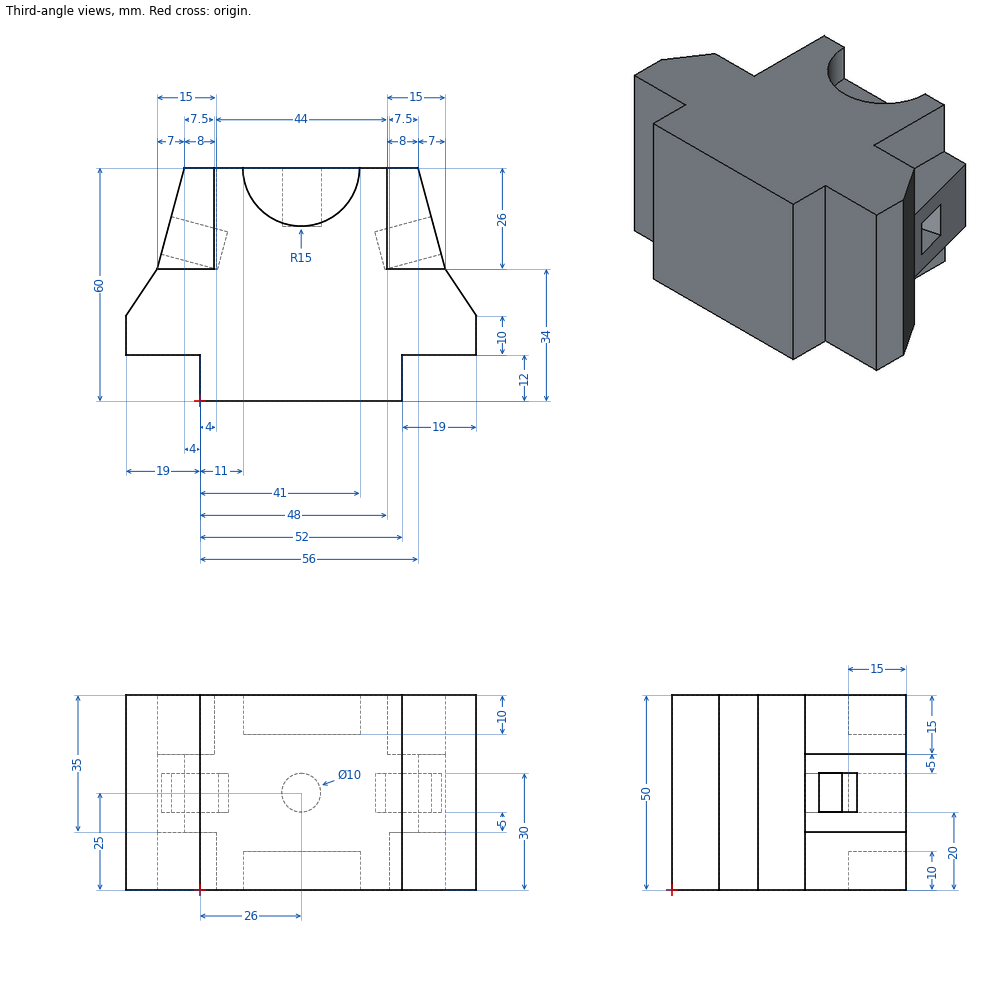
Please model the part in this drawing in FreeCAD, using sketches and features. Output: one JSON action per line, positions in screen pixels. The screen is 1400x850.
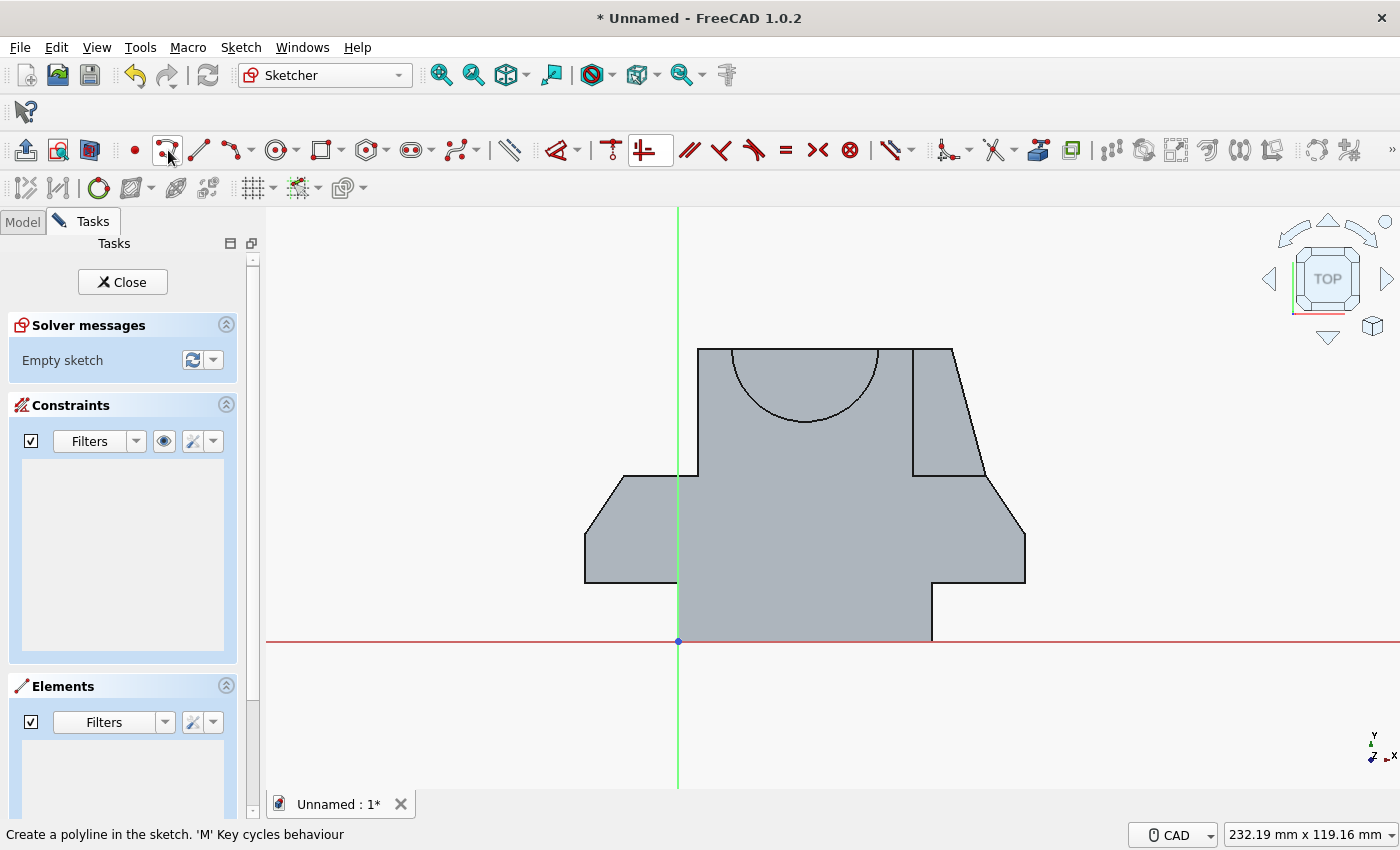
{"action": "left_click", "coordinate": [698, 476]}
{"action": "left_click", "coordinate": [698, 349]}
{"action": "left_click", "coordinate": [659, 349]}
{"action": "left_click", "coordinate": [624, 476]}
{"action": "left_click", "coordinate": [698, 477]}
{"action": "key", "text": "Escape"}
{"action": "key", "text": "Escape"}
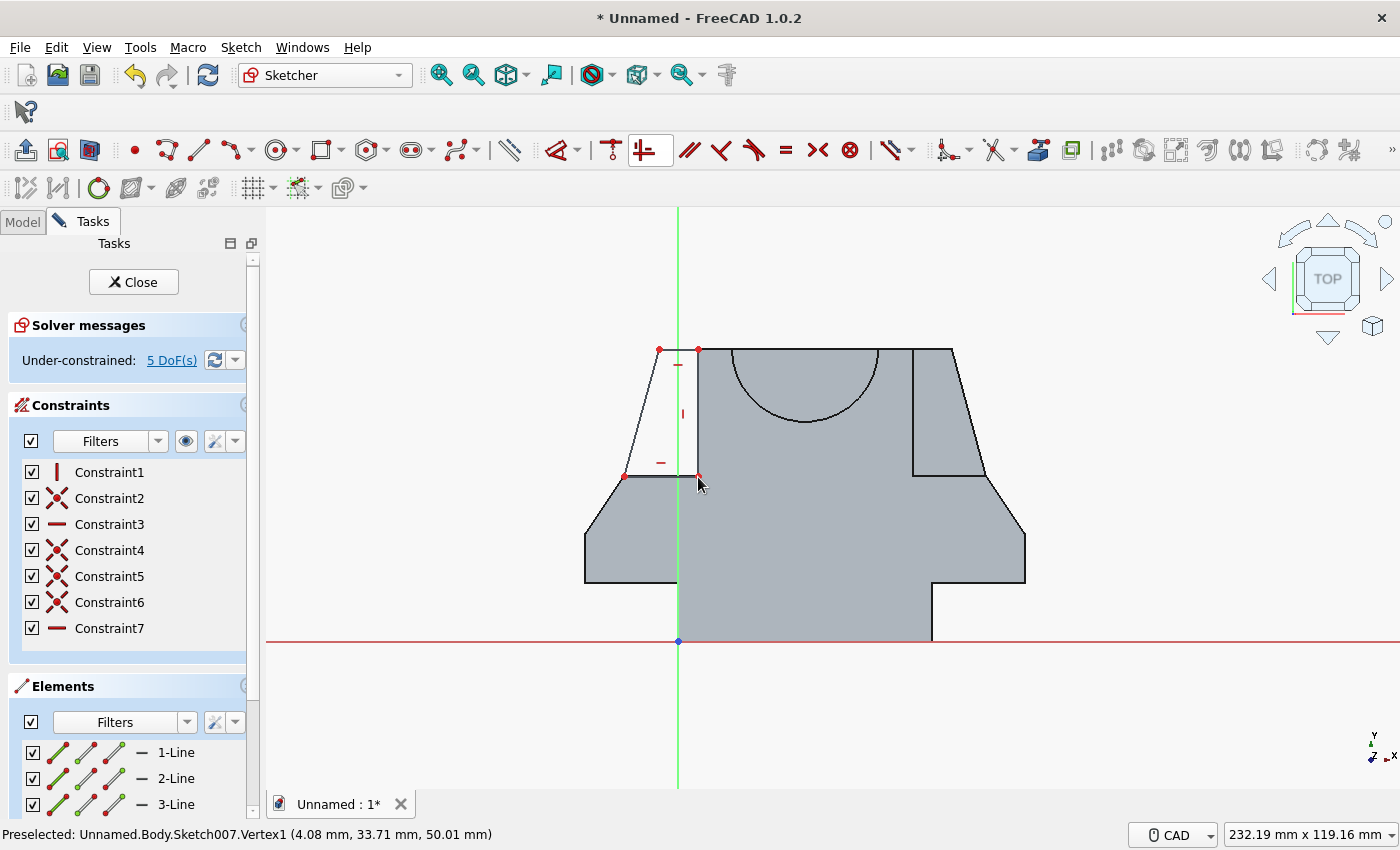
{"action": "left_click", "coordinate": [556, 150]}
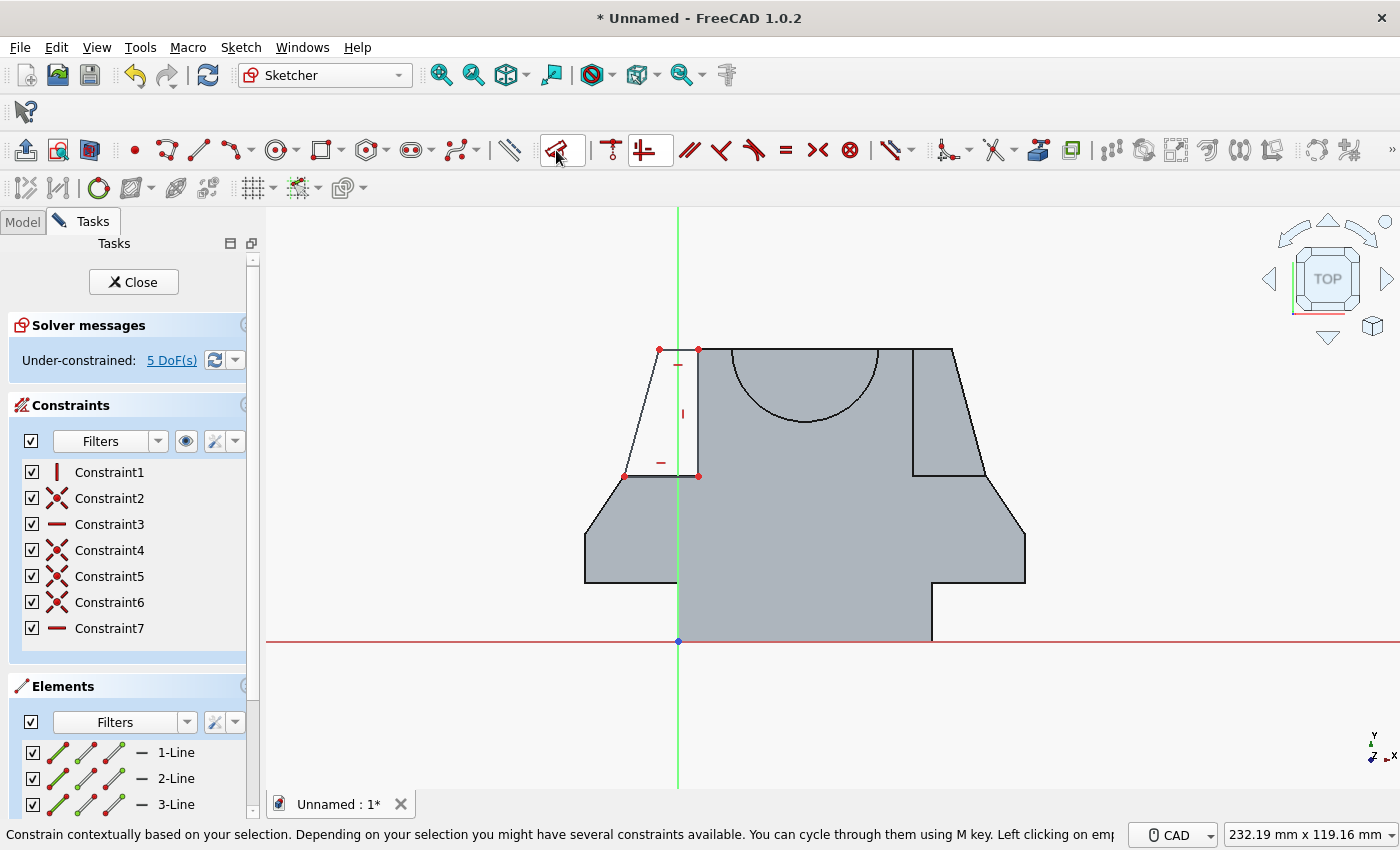
{"action": "left_click", "coordinate": [675, 350]}
{"action": "left_click", "coordinate": [665, 316]}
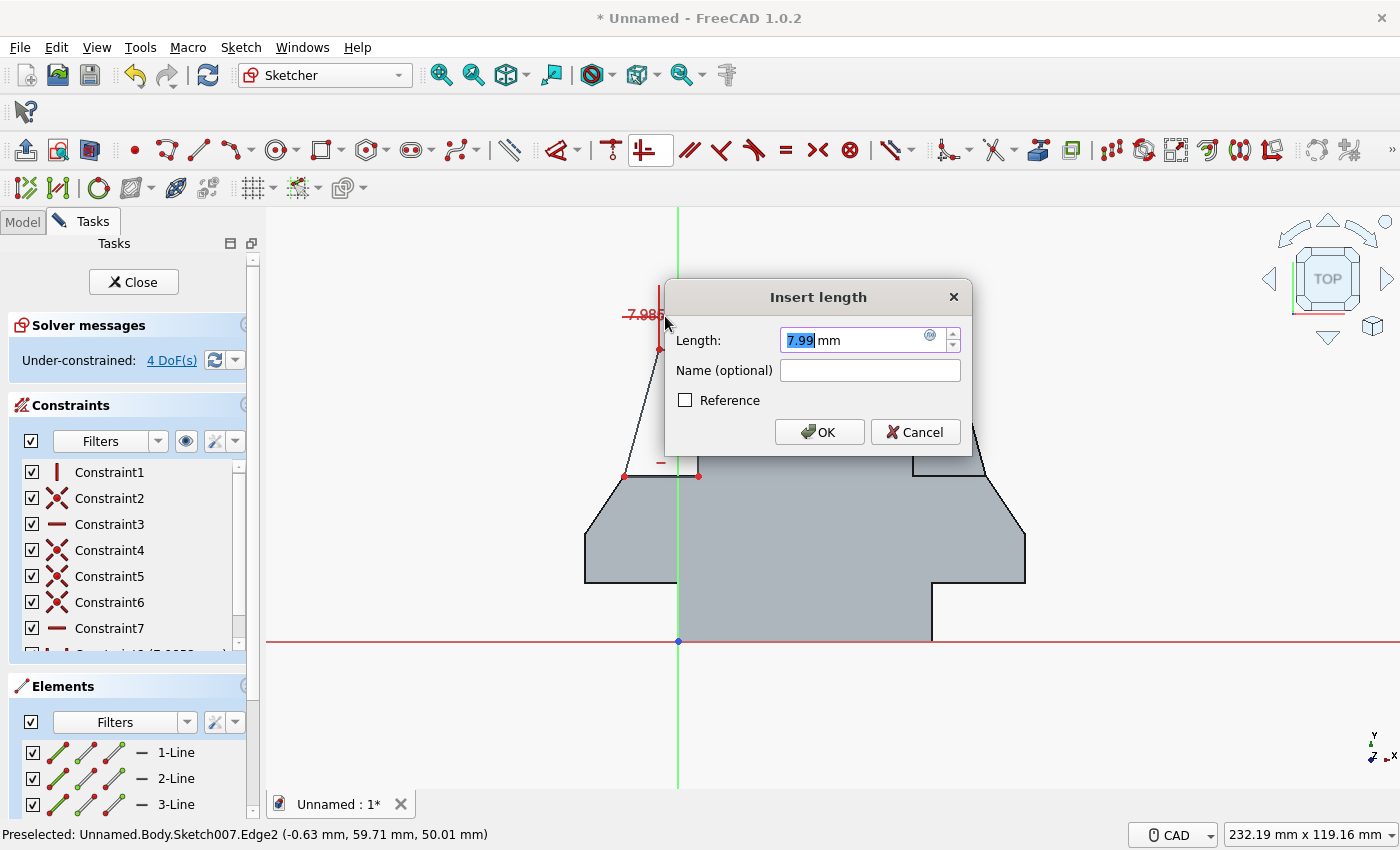
{"action": "type", "text": "8"}
{"action": "key", "text": "Return"}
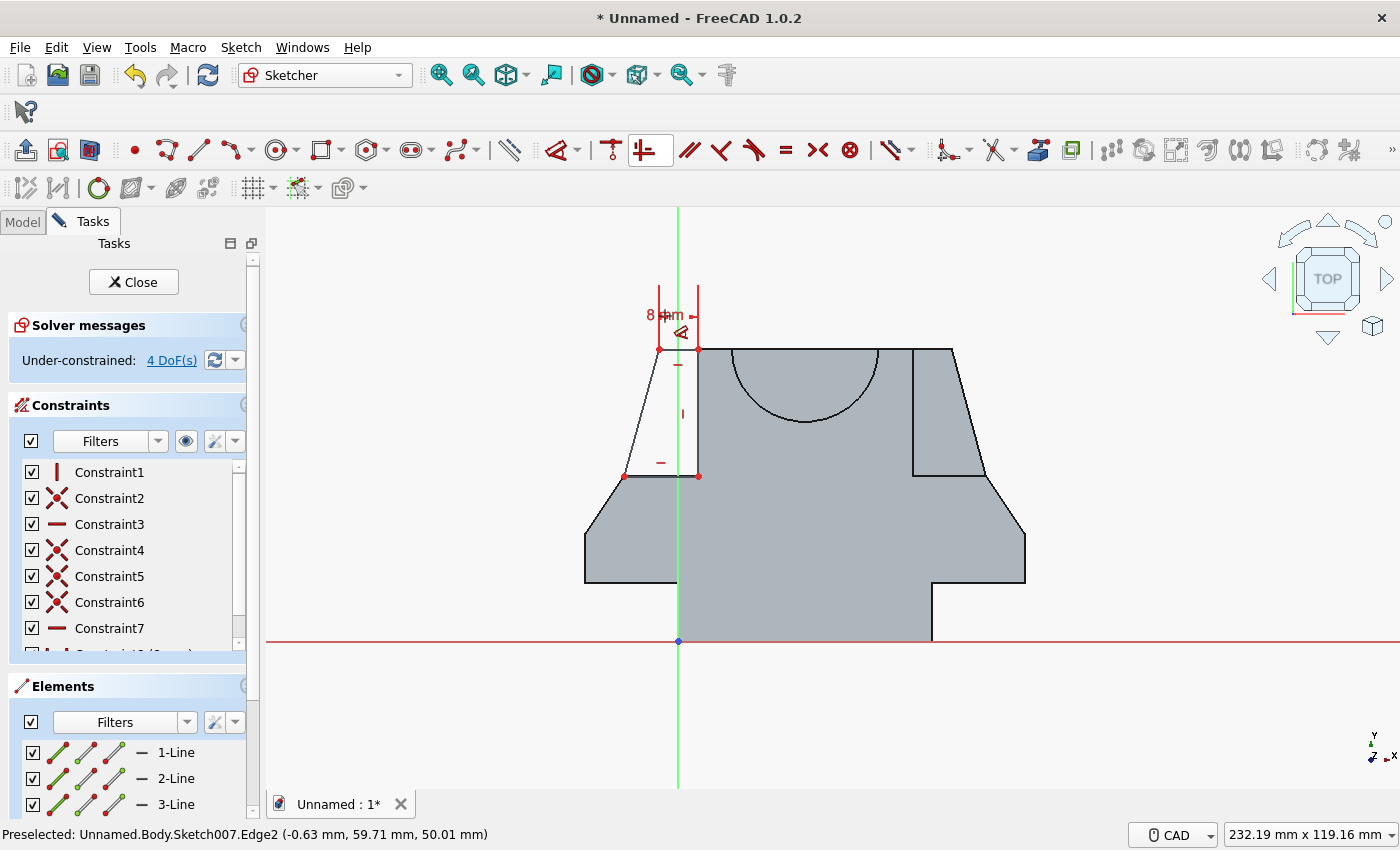
{"action": "left_click", "coordinate": [698, 439]}
{"action": "left_click", "coordinate": [732, 414]}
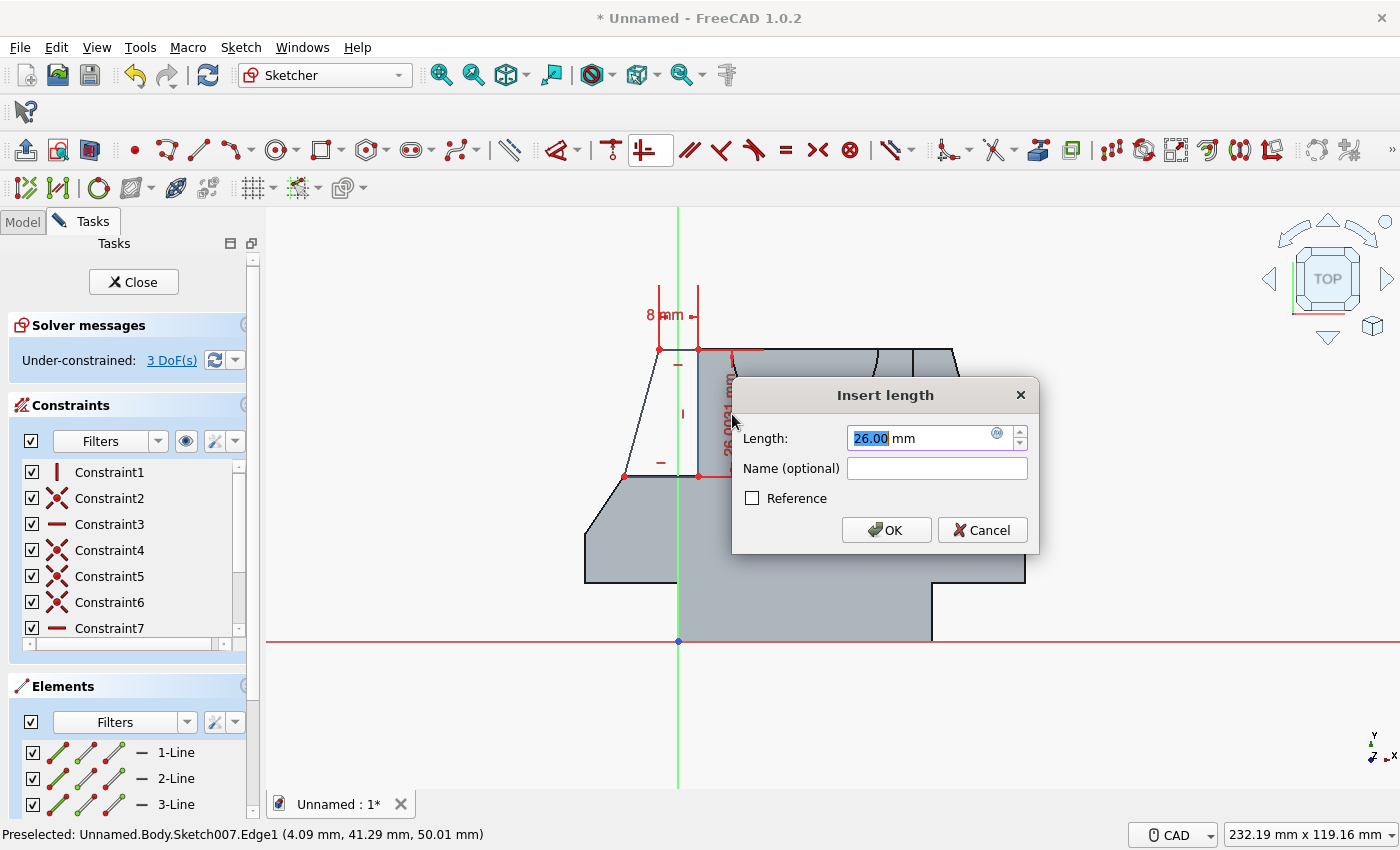
{"action": "type", "text": "26"}
{"action": "key", "text": "Return"}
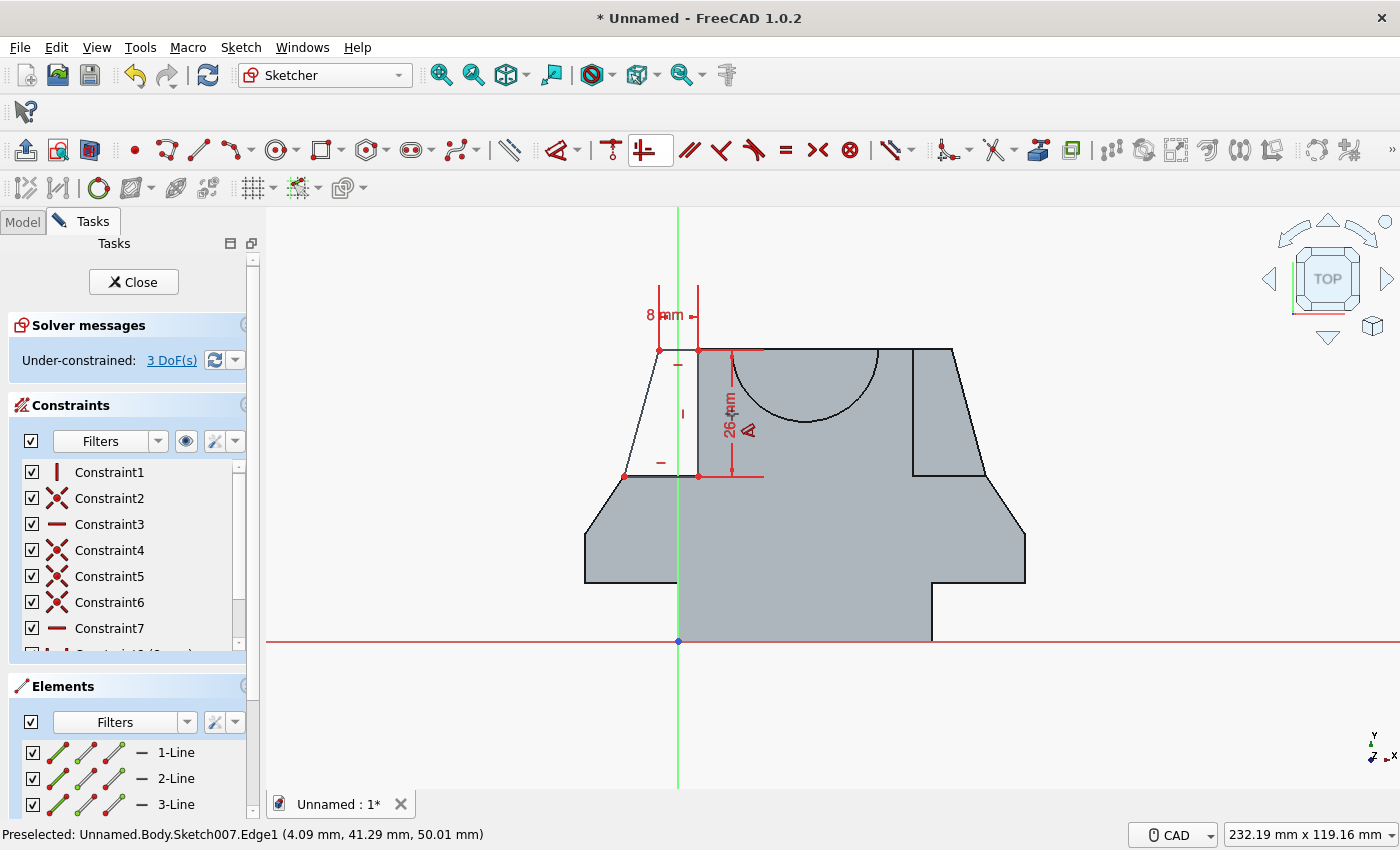
{"action": "left_click", "coordinate": [646, 477]}
{"action": "left_click", "coordinate": [661, 443]}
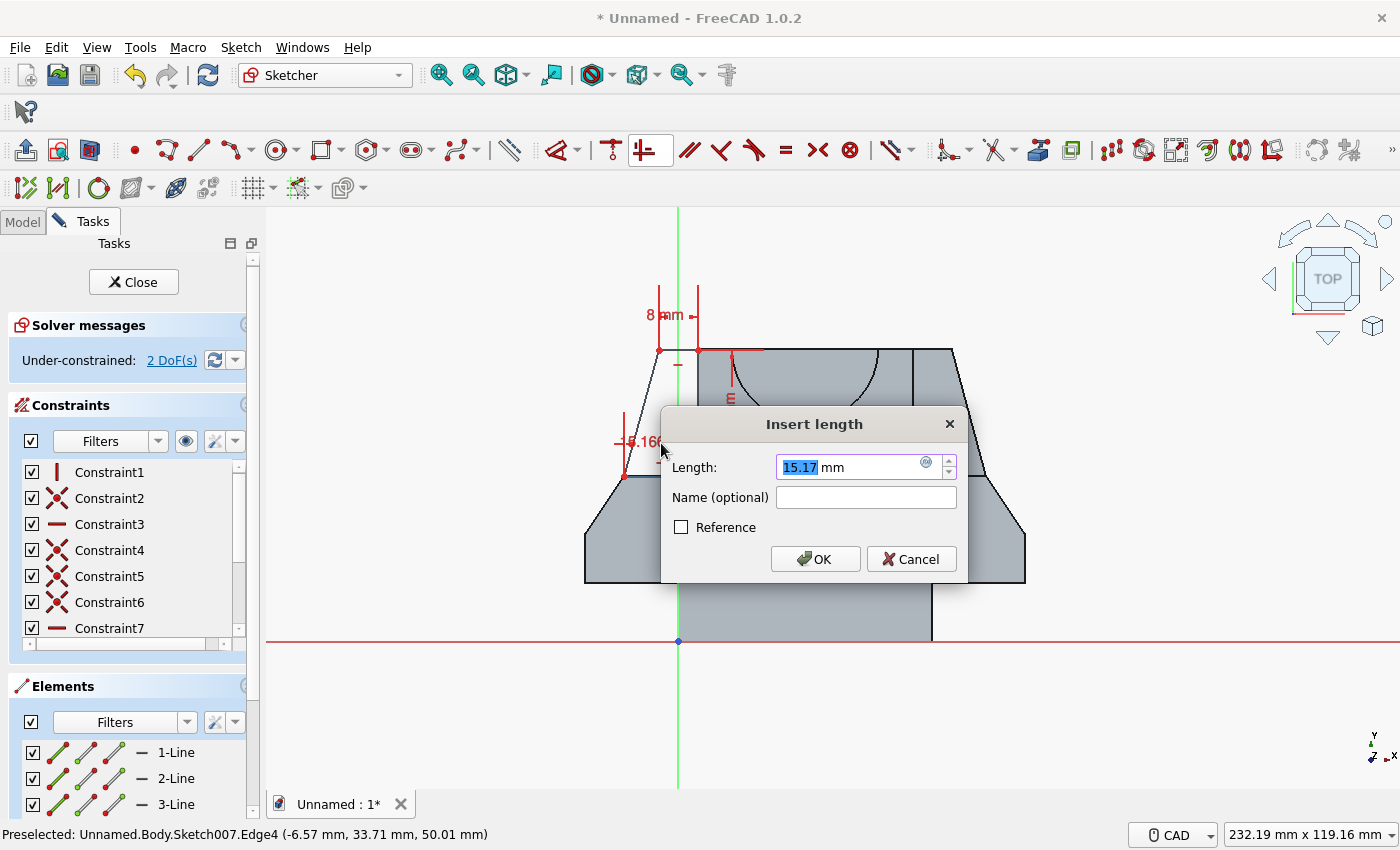
{"action": "type", "text": "15"}
{"action": "key", "text": "Return"}